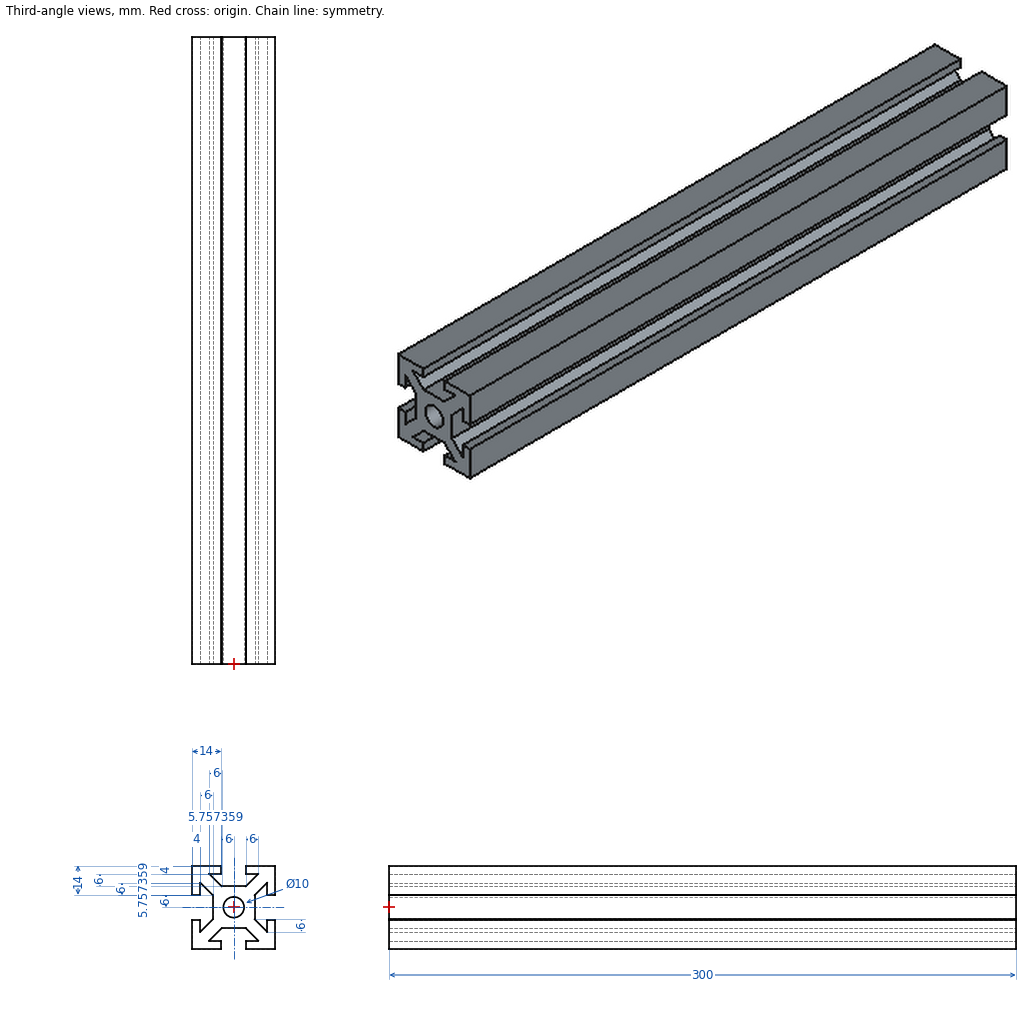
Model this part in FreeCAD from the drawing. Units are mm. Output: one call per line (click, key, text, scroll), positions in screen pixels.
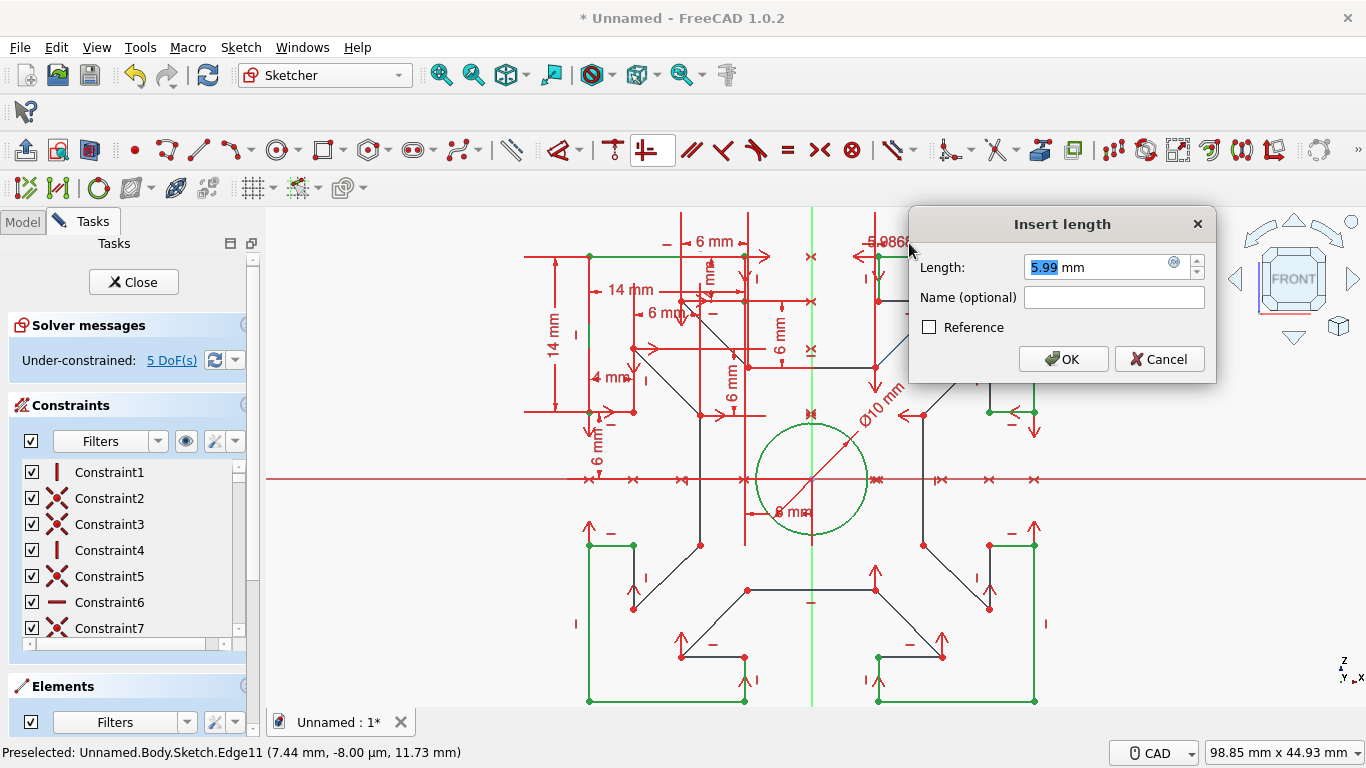
text(6)
key(Return)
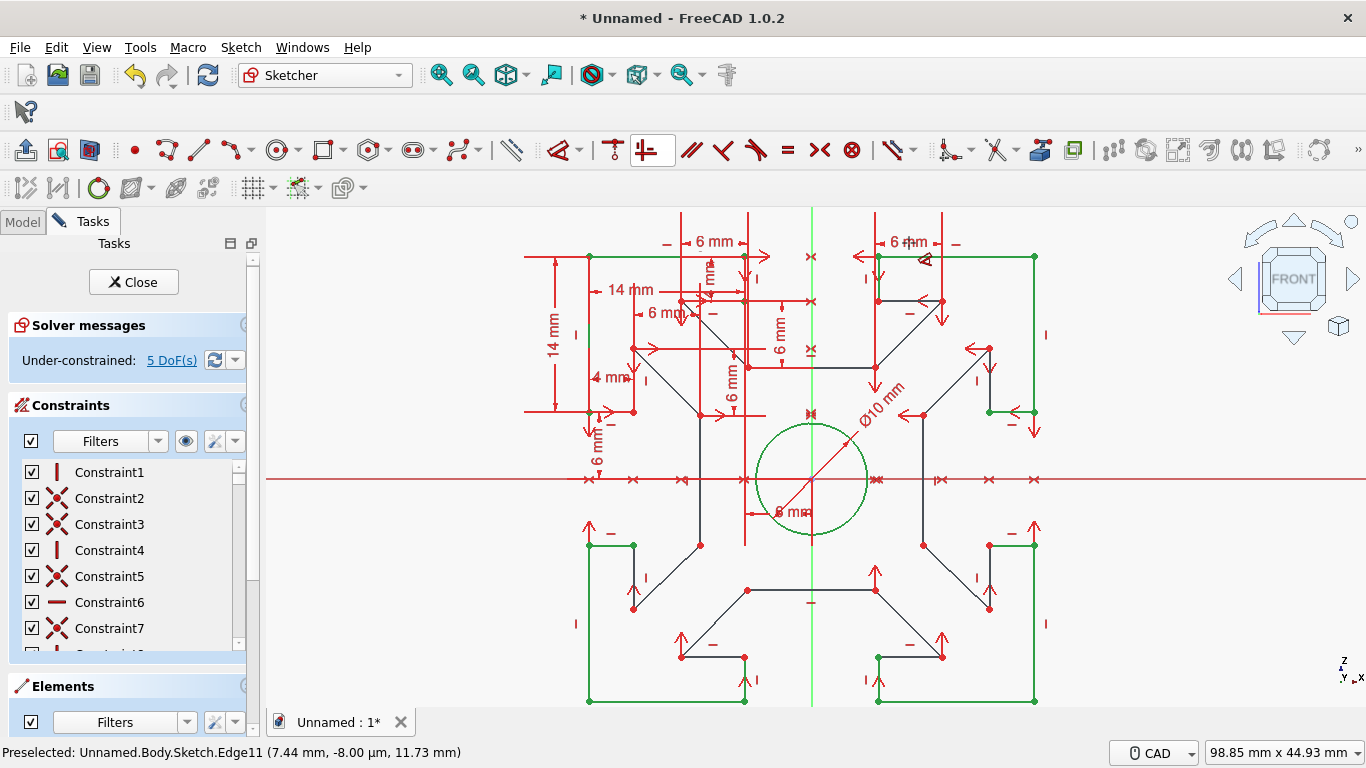
click(943, 564)
click(889, 577)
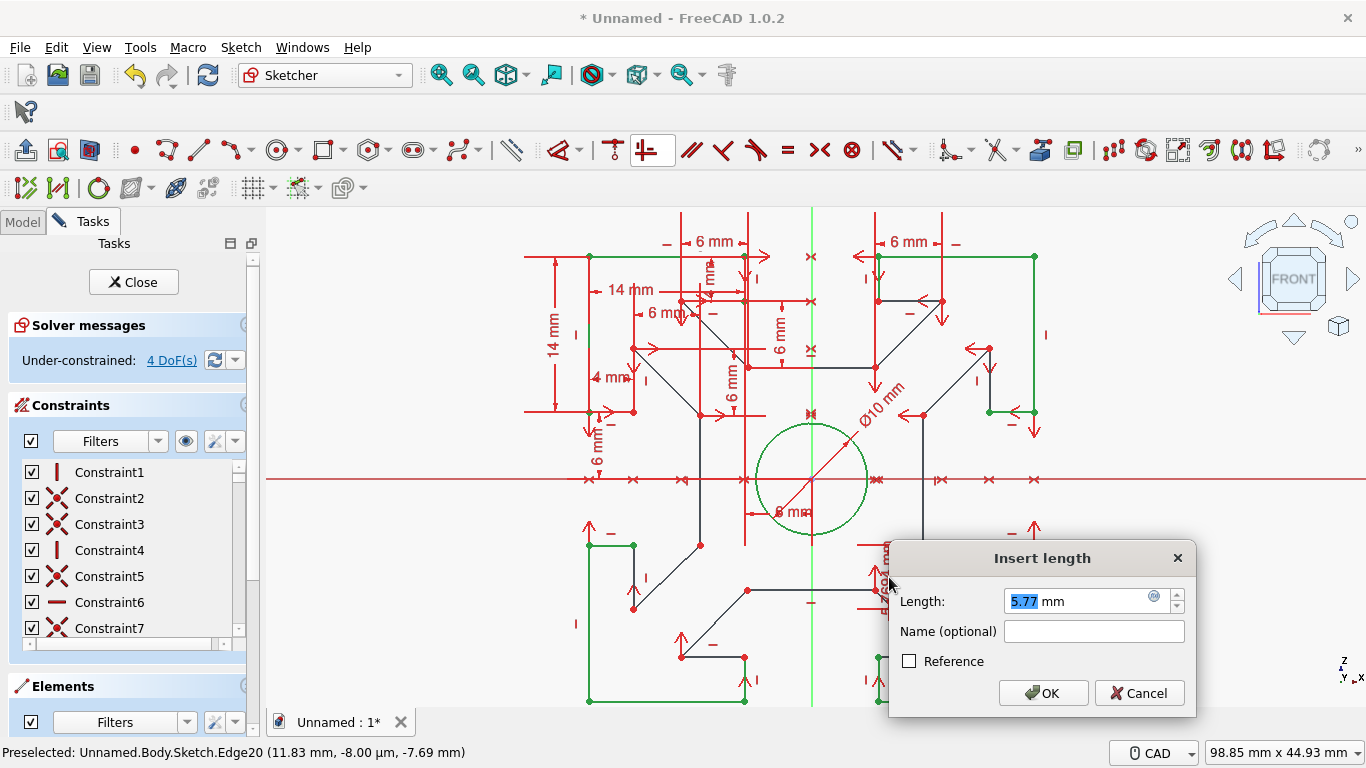
text(6)
key(Return)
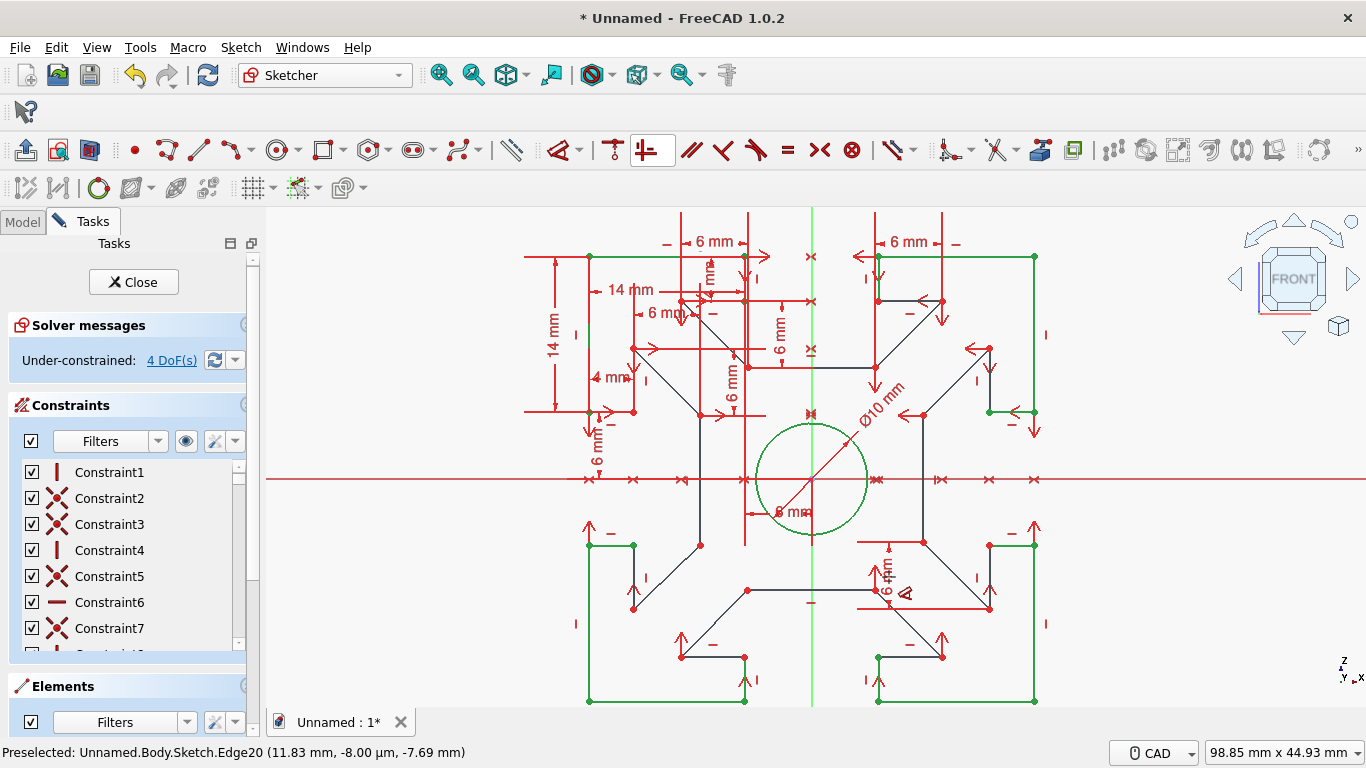
click(727, 610)
click(714, 556)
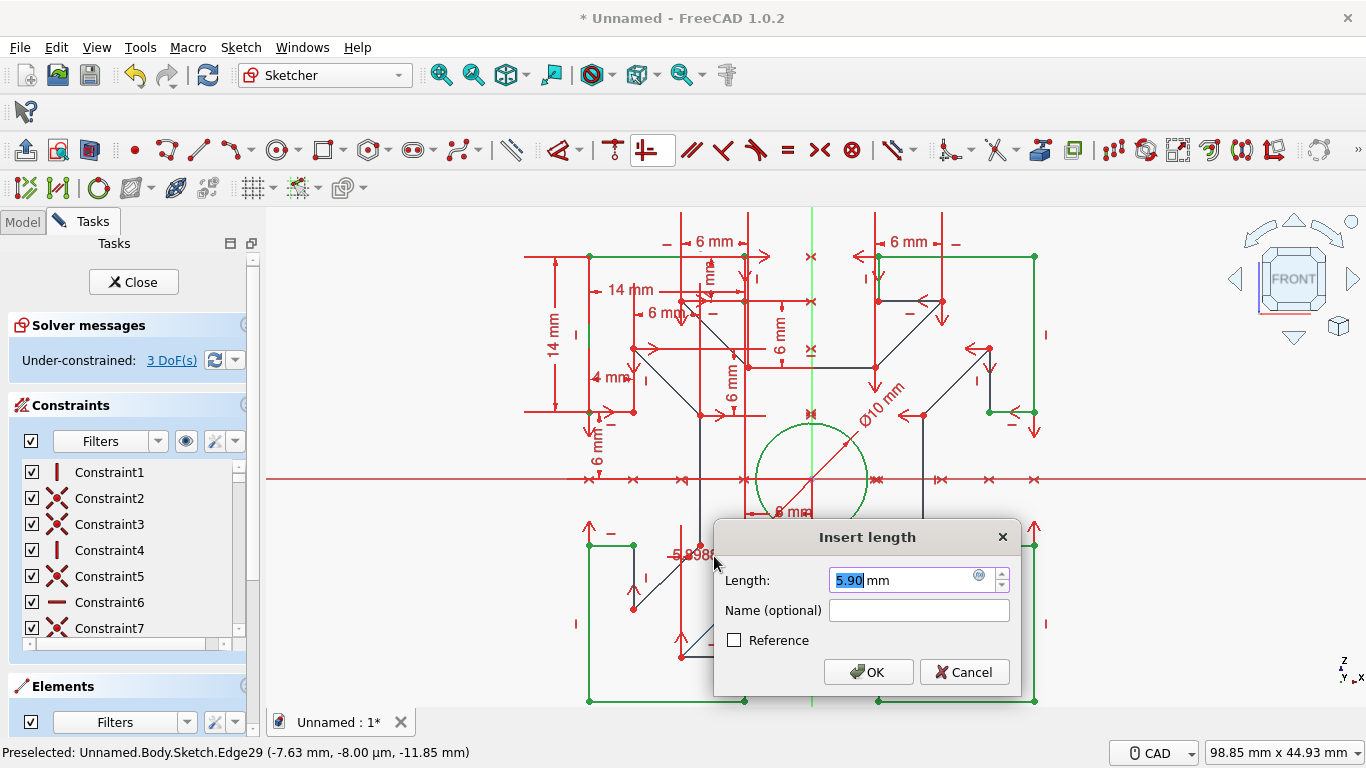
text(6)
key(Return)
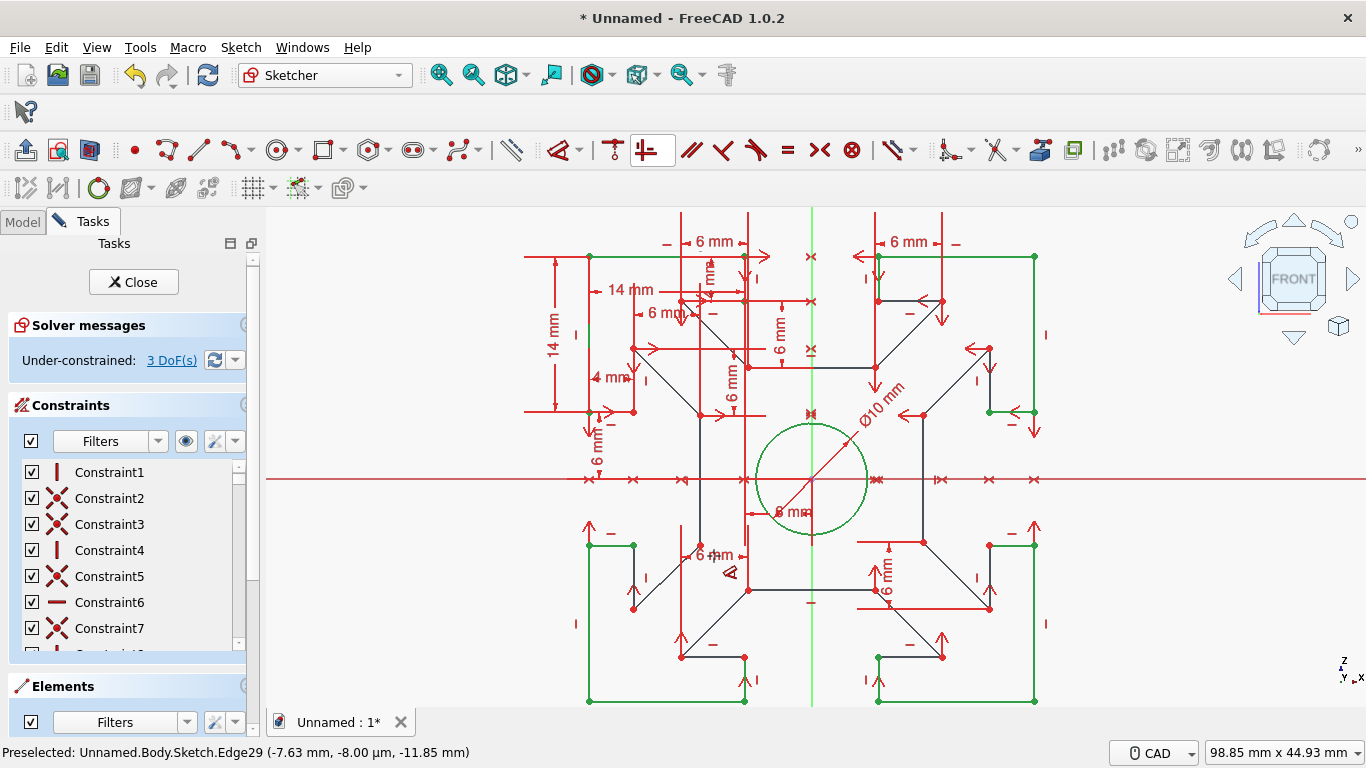
click(654, 590)
click(734, 577)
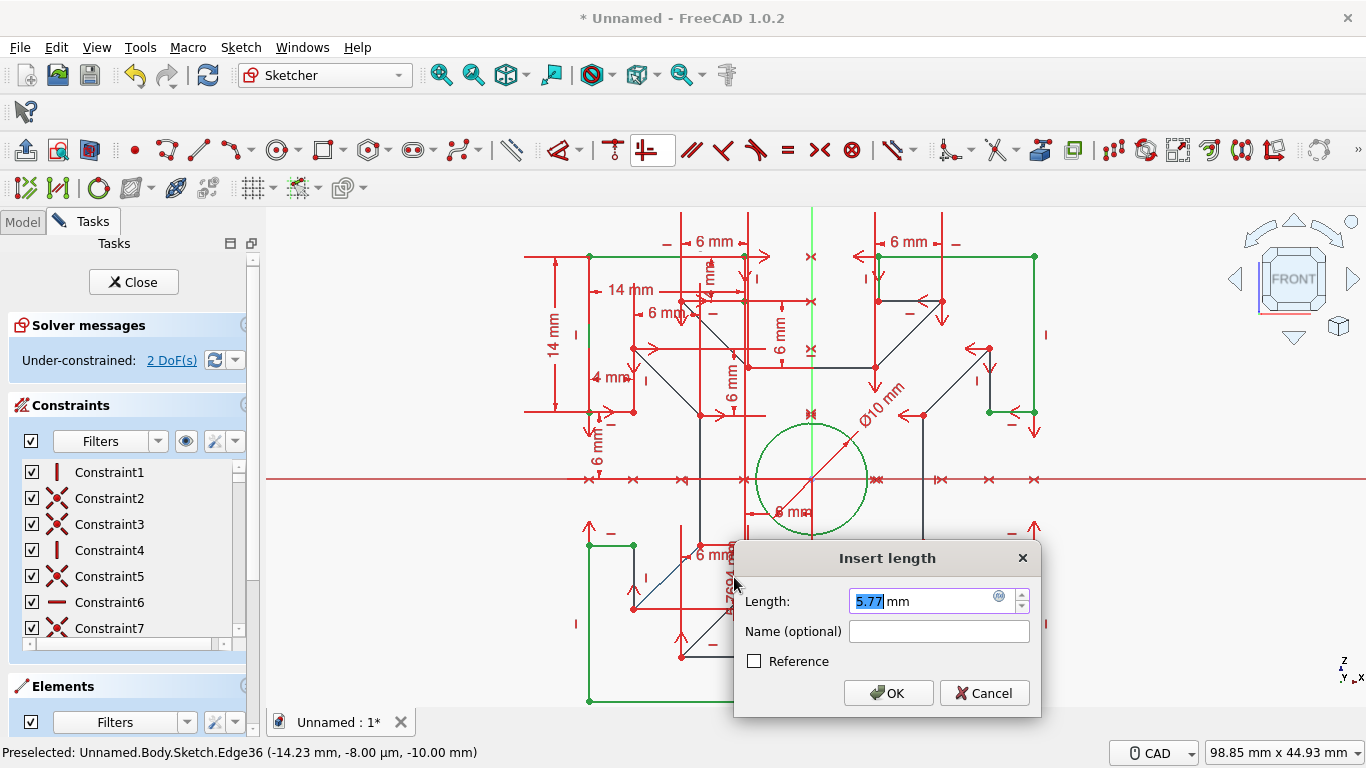
text(6)
key(Return)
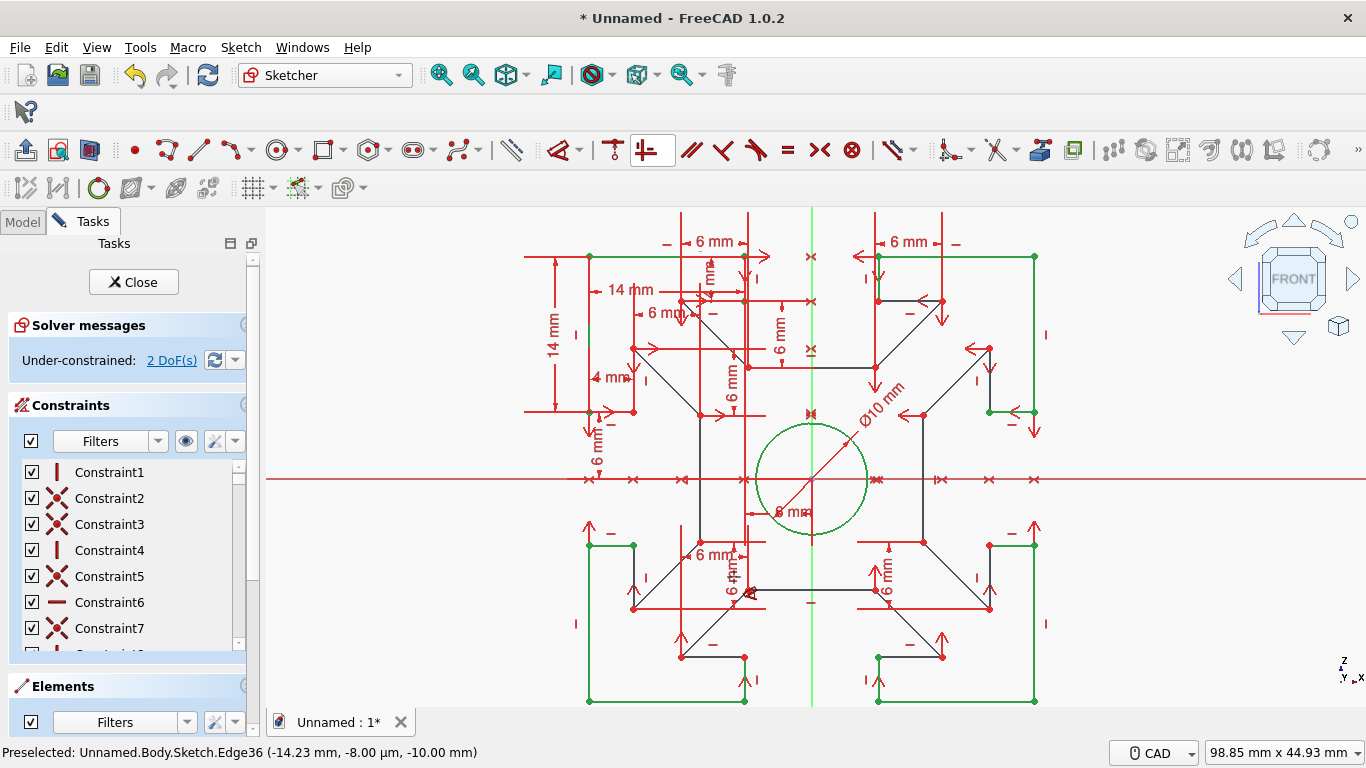
click(634, 368)
click(576, 403)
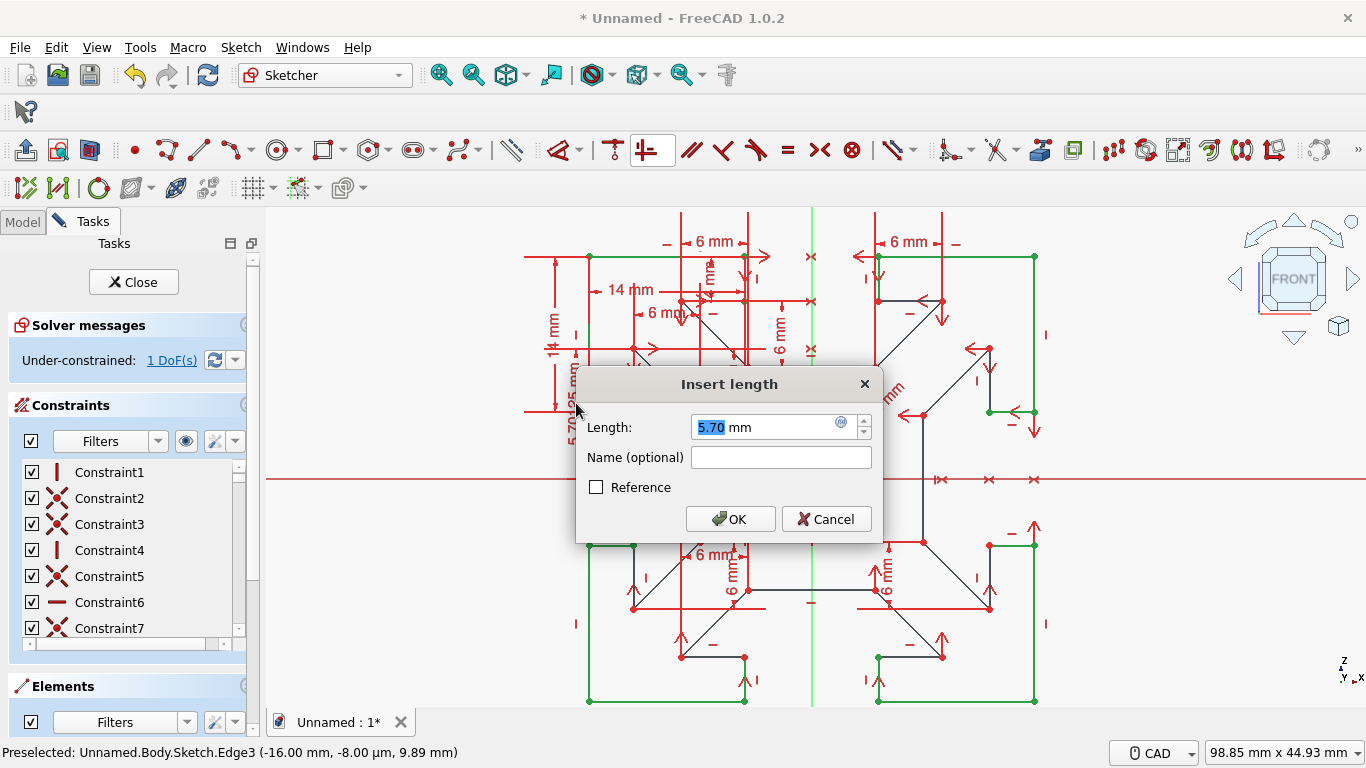
text(5.757359)
key(Return)